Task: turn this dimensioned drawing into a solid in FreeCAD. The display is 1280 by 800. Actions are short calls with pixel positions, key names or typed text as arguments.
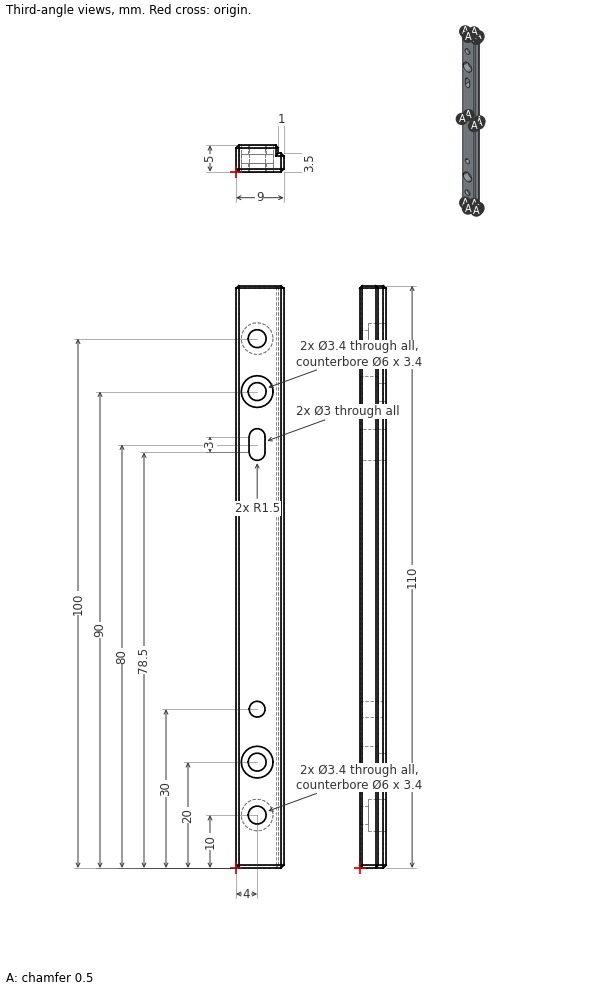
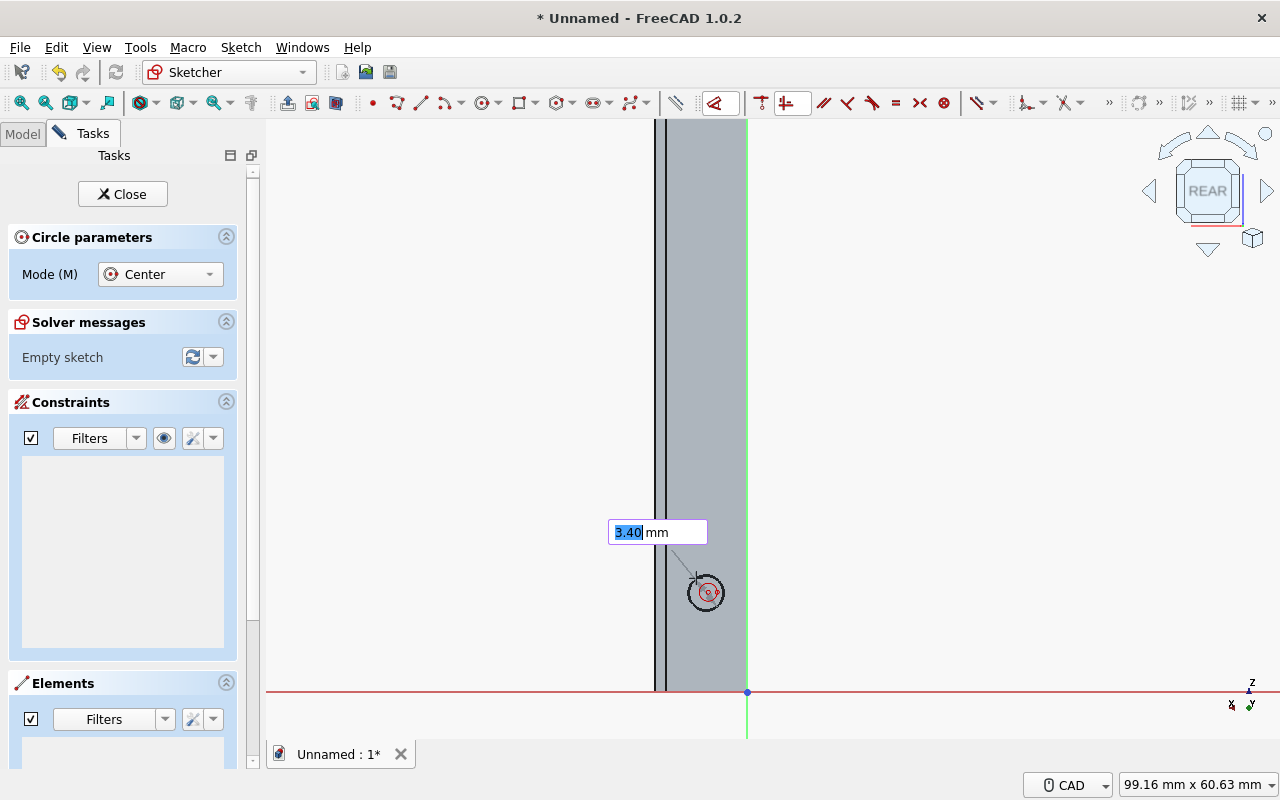
click(694, 578)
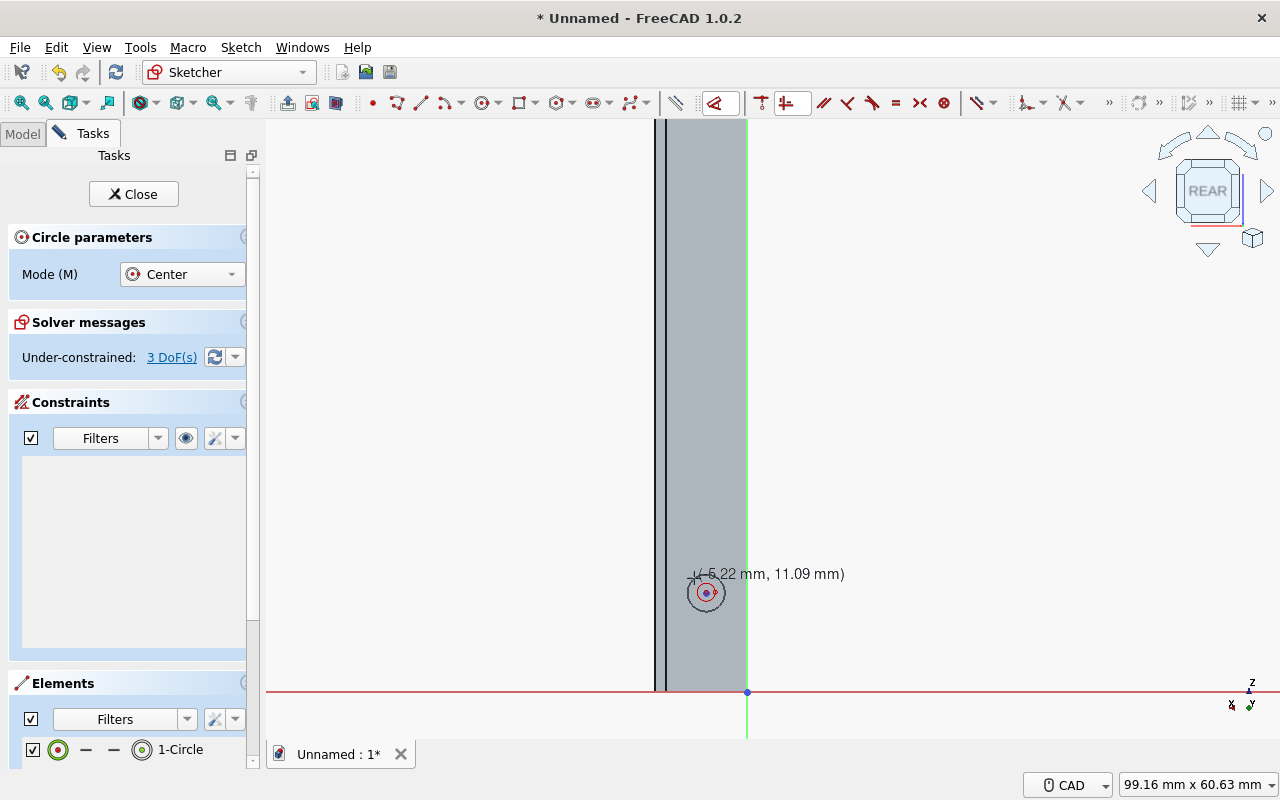
scroll(696, 578, down, 5)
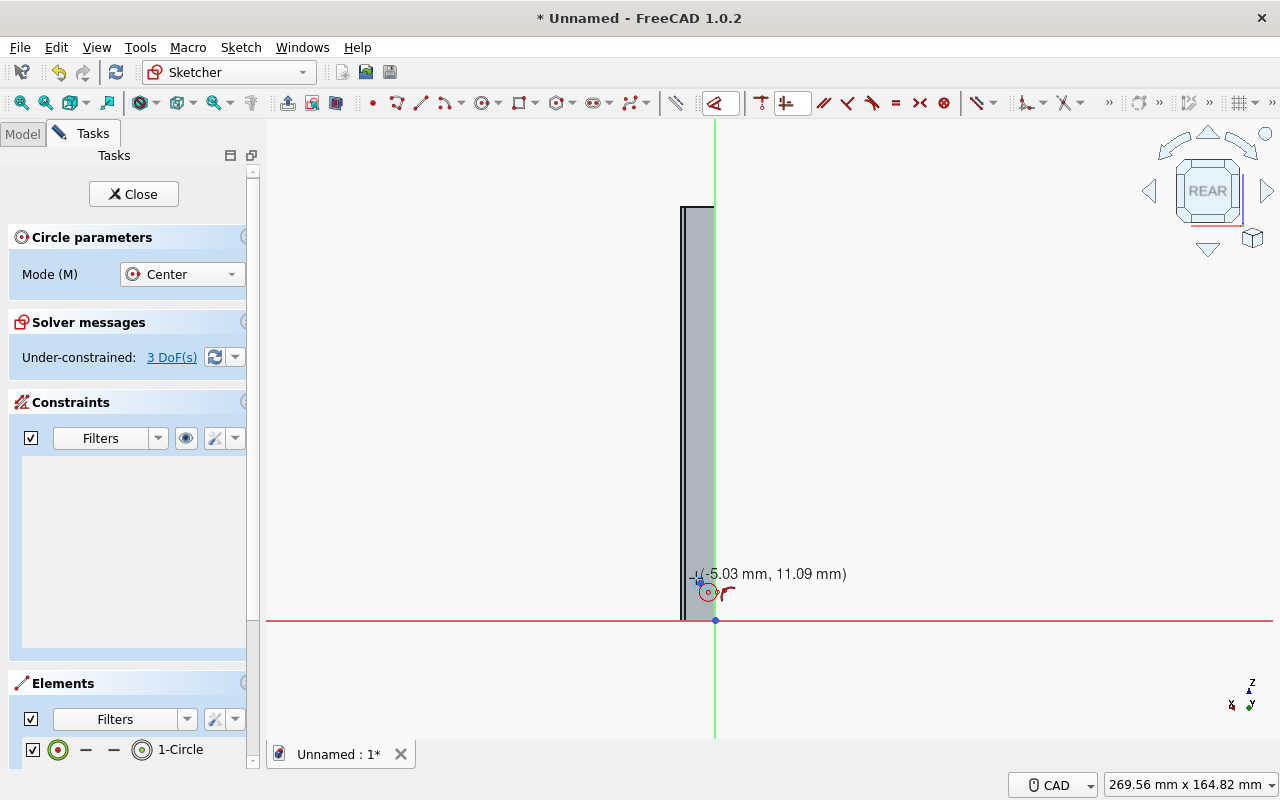
scroll(700, 244, up, 7)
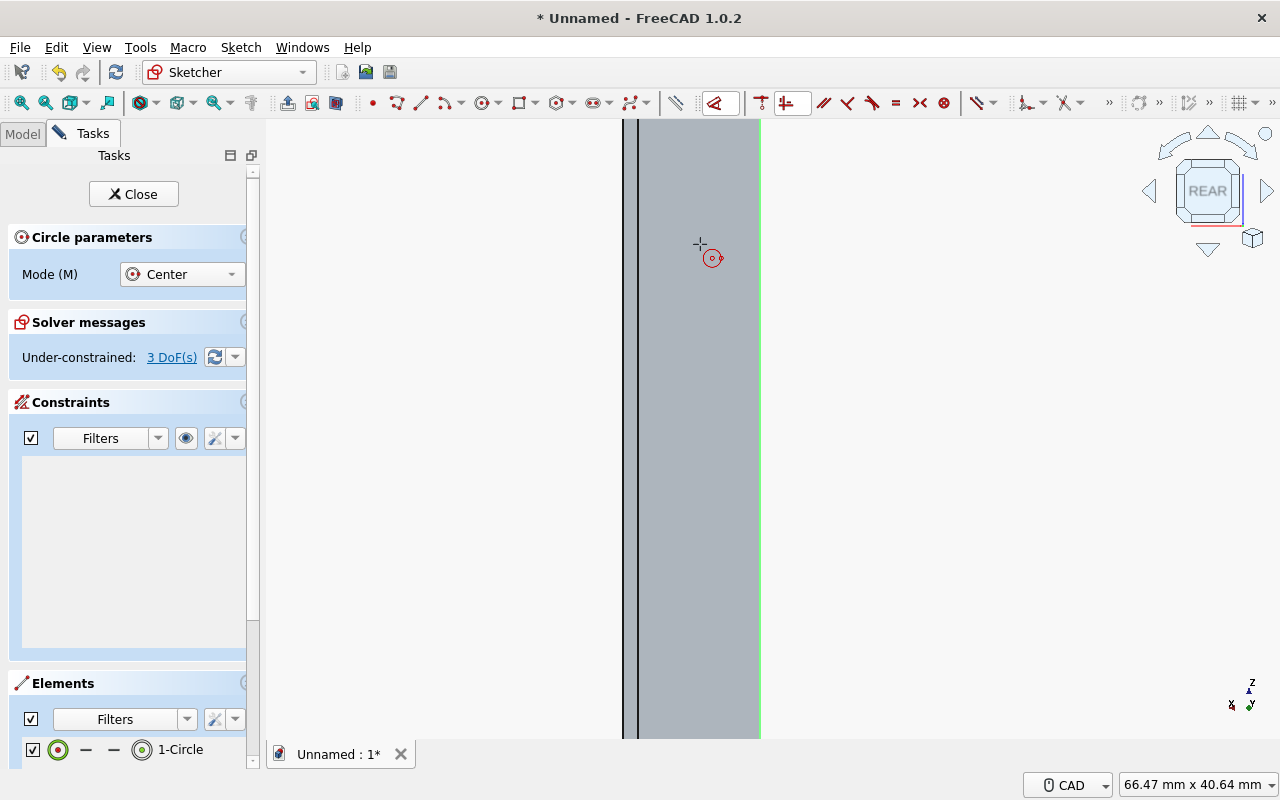
scroll(700, 244, down, 7)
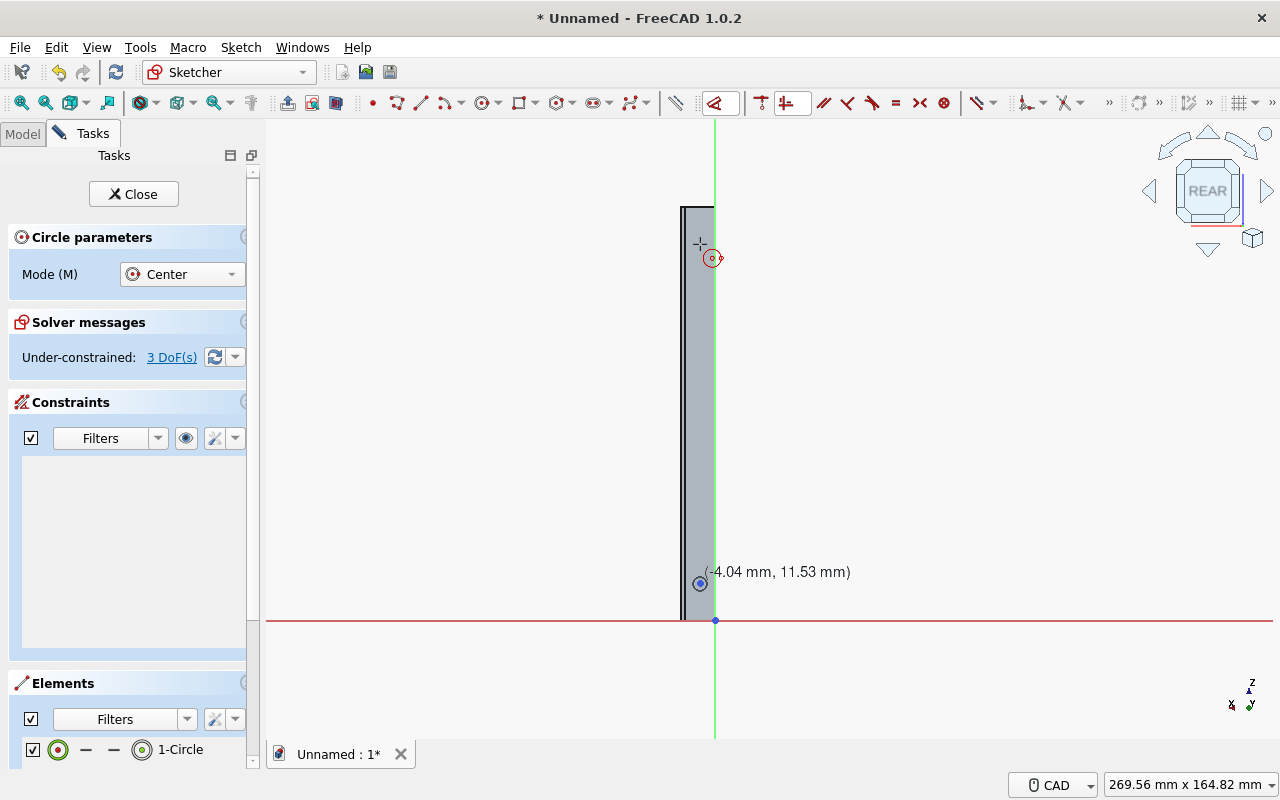
click(700, 244)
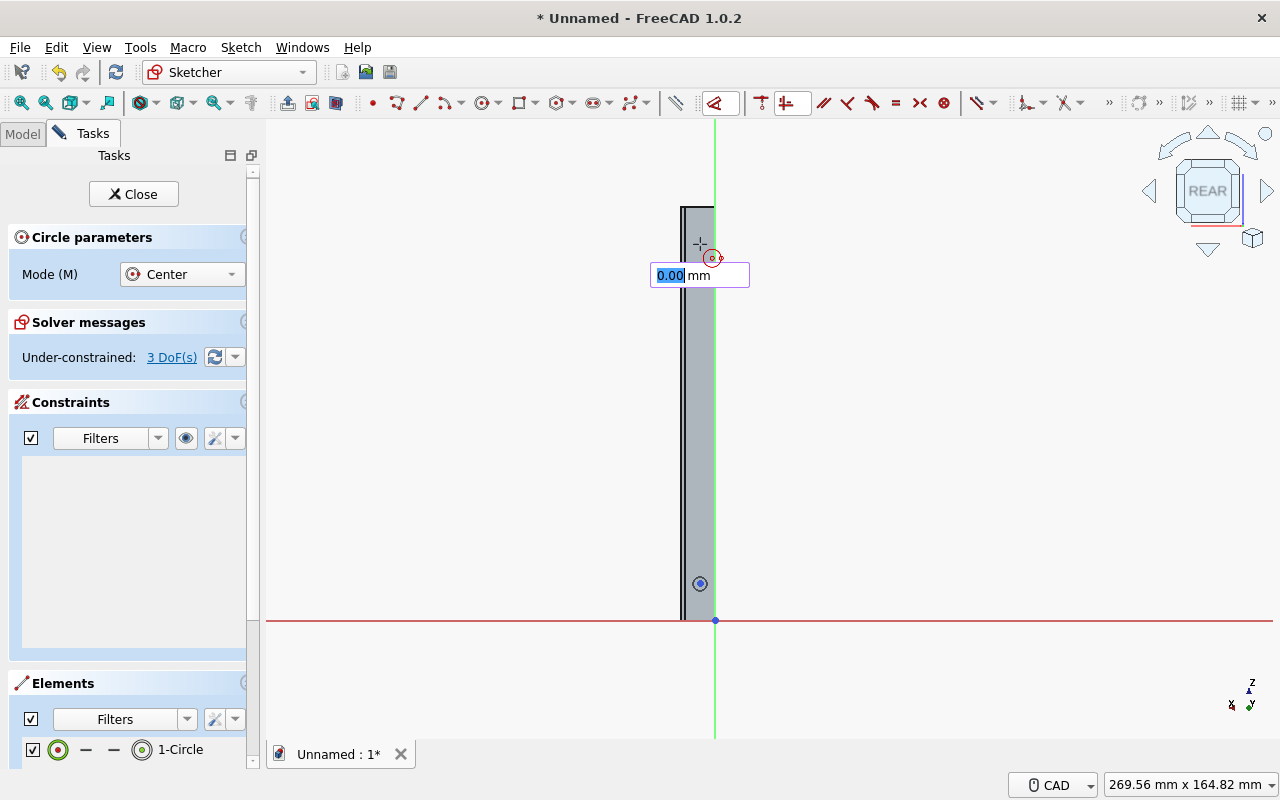
scroll(696, 240, up, 5)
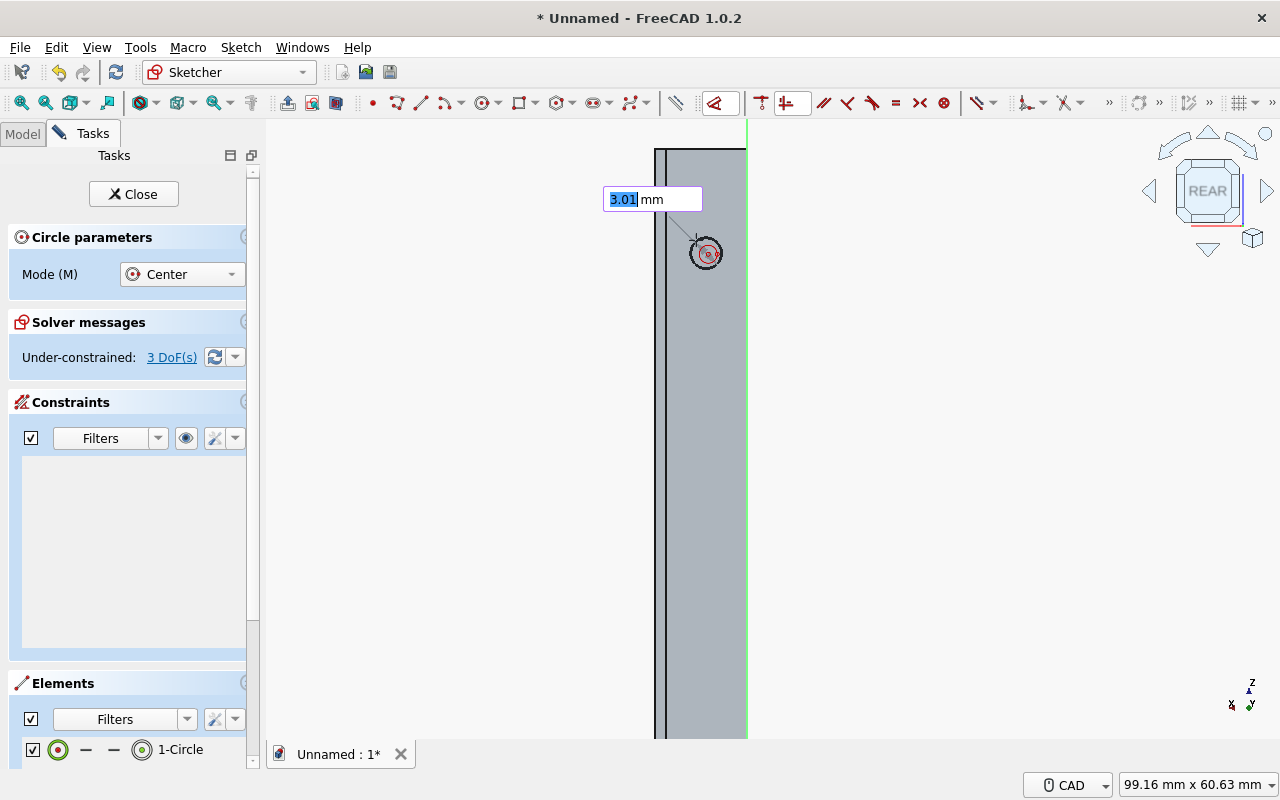
click(694, 239)
key(Escape)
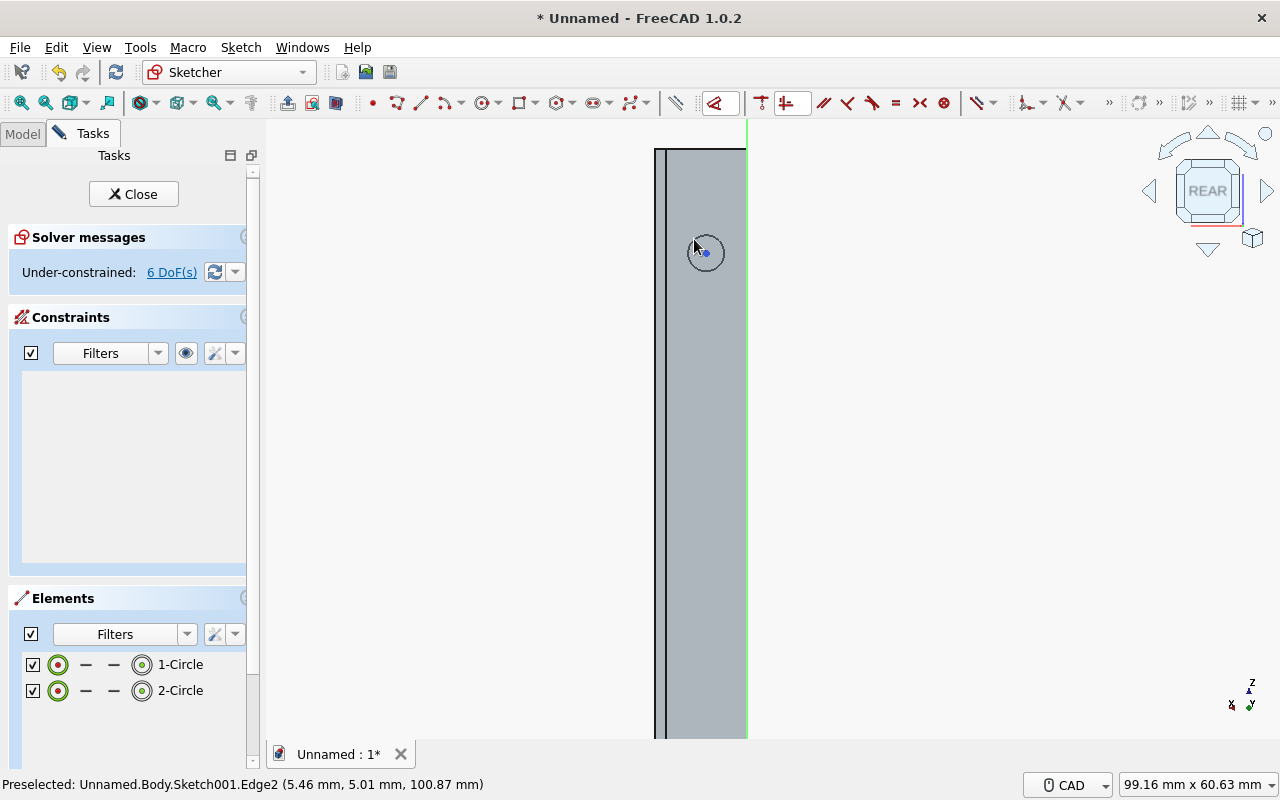
scroll(696, 240, down, 5)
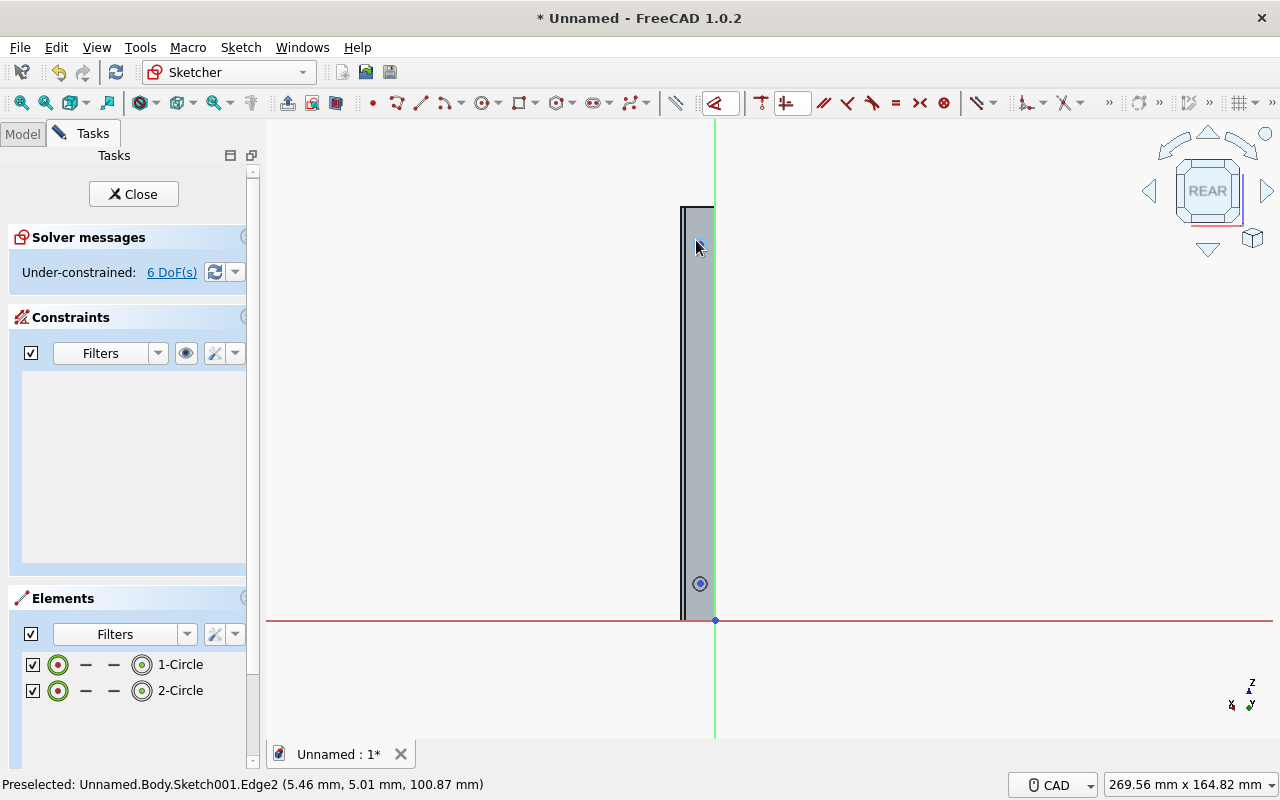
scroll(705, 579, up, 4)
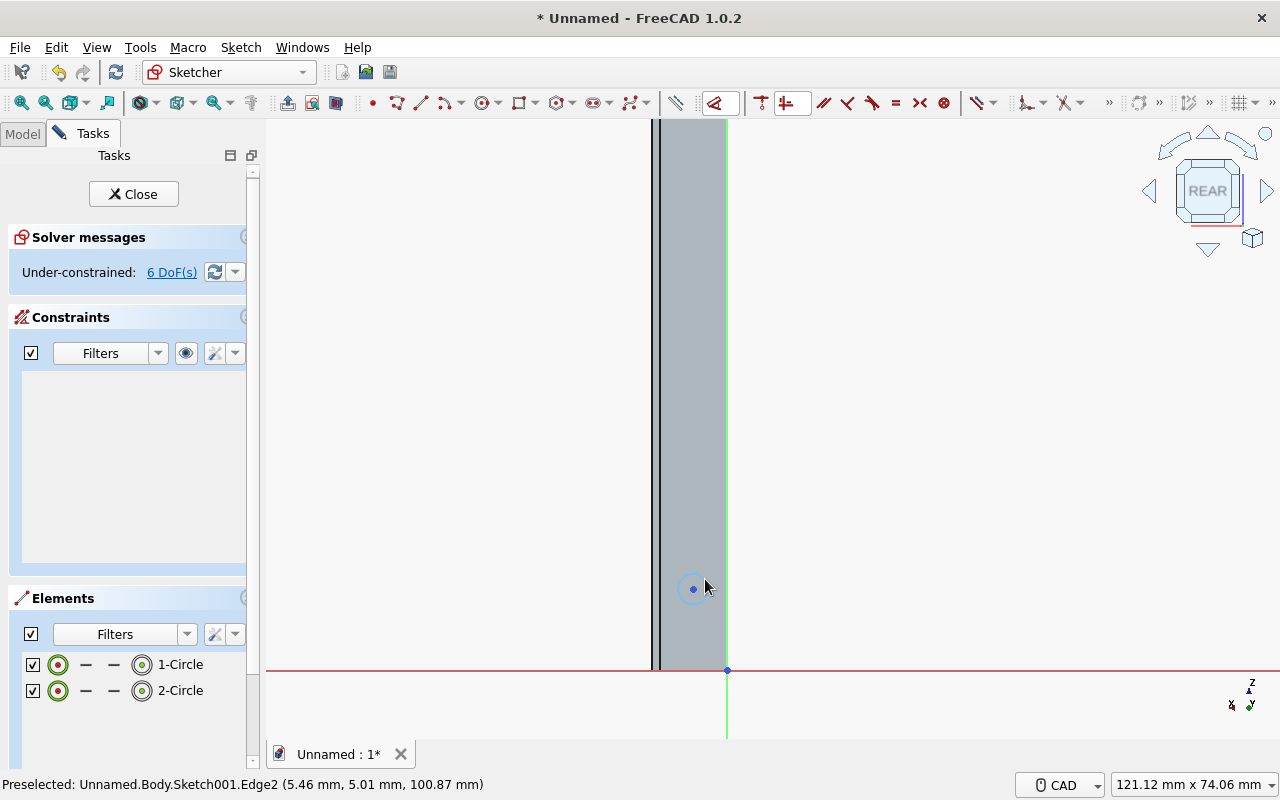
click(704, 578)